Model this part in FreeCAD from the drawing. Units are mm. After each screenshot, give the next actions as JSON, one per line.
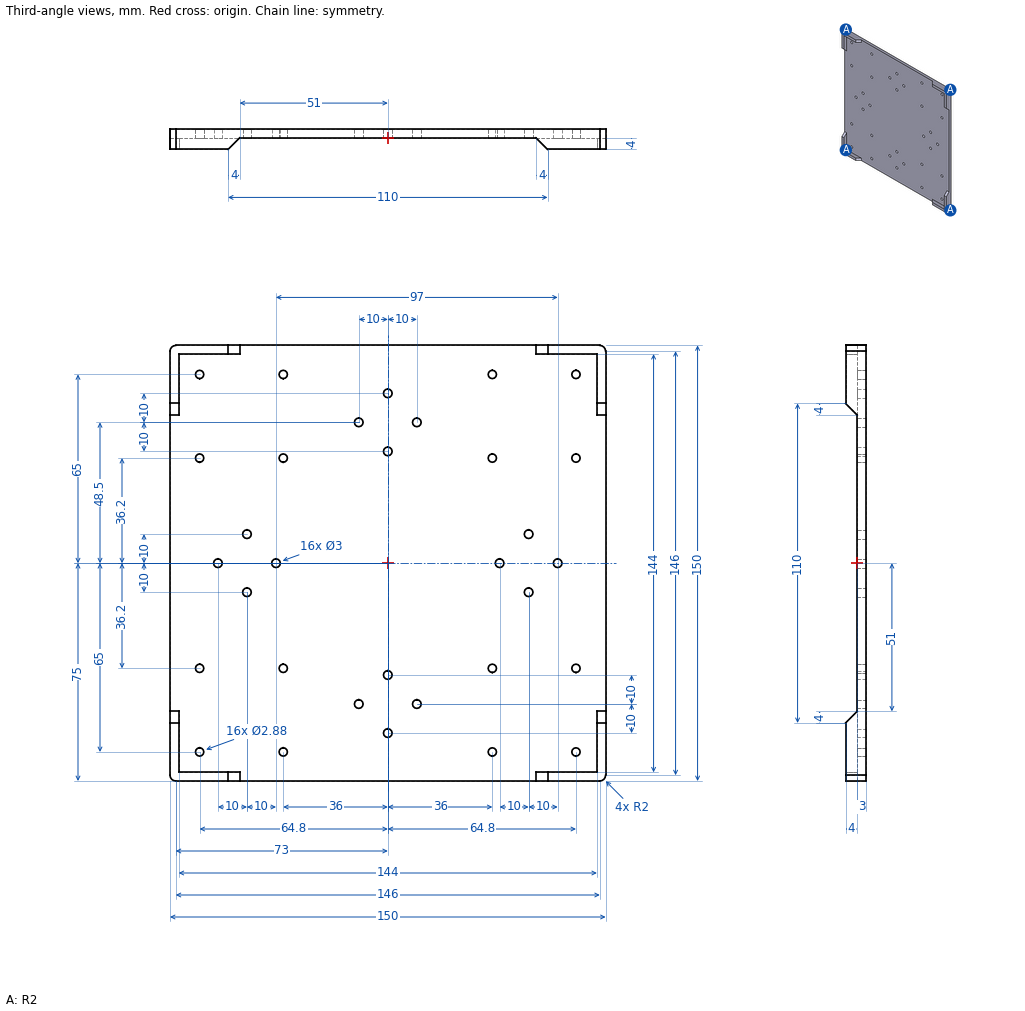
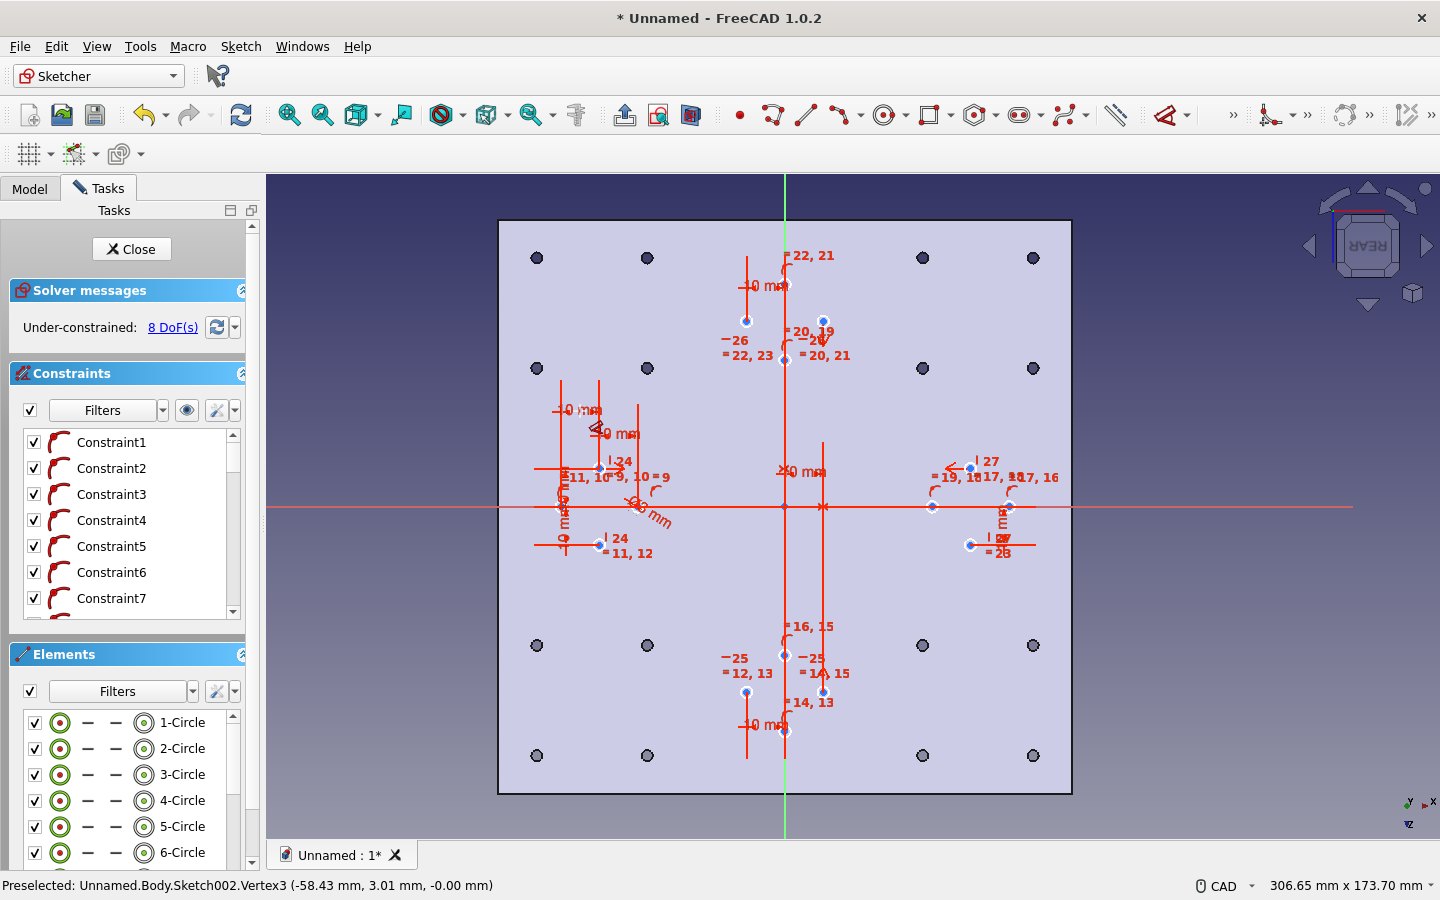
{"action": "left_click", "coordinate": [747, 692]}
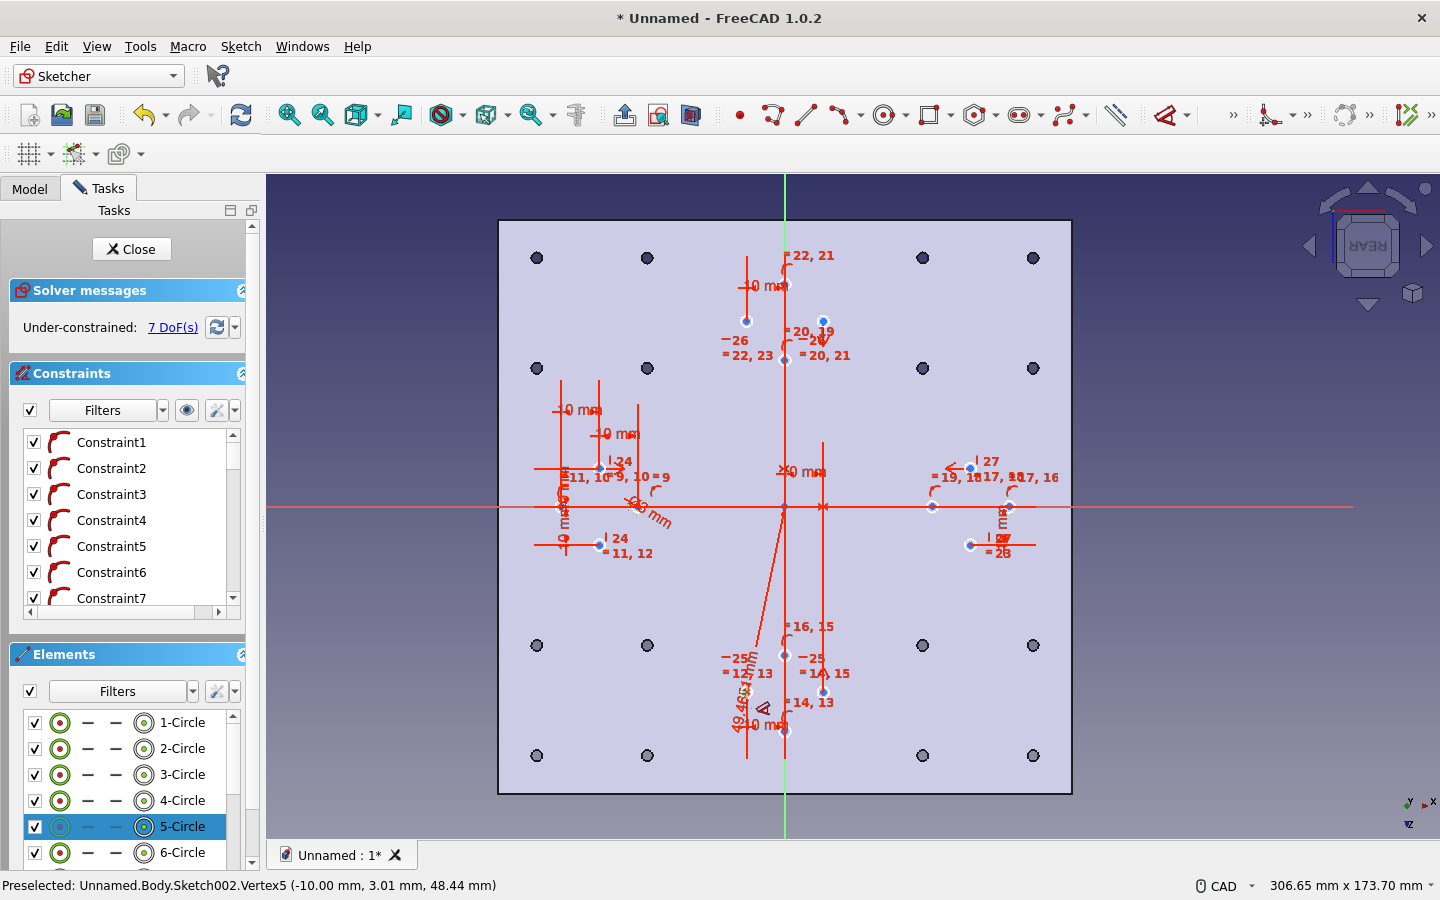
{"action": "left_click", "coordinate": [785, 732]}
{"action": "left_click", "coordinate": [713, 703]}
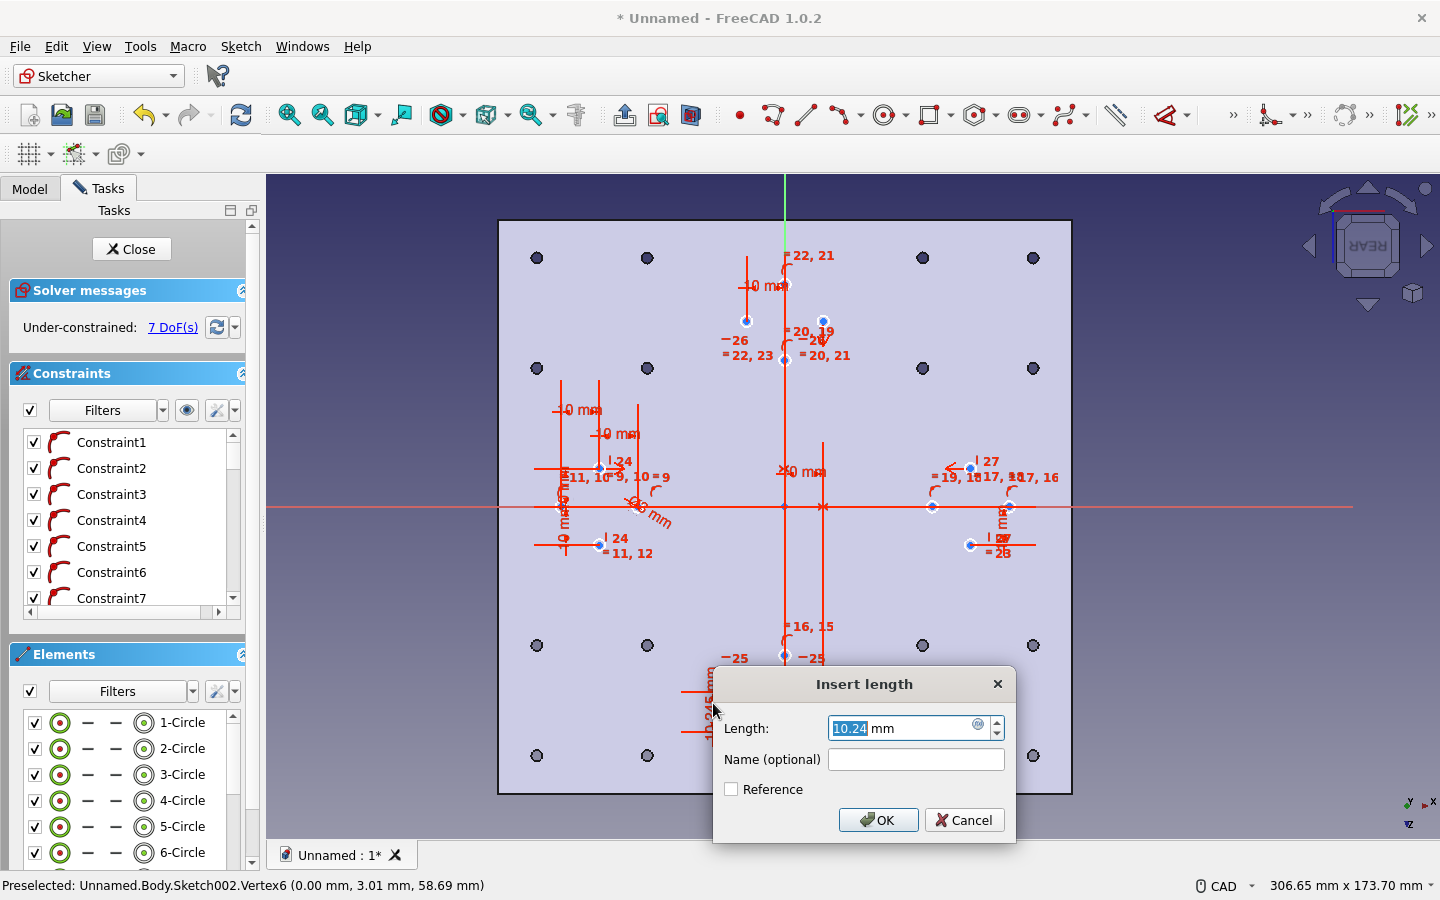
{"action": "type", "text": "10"}
{"action": "key", "text": "Return"}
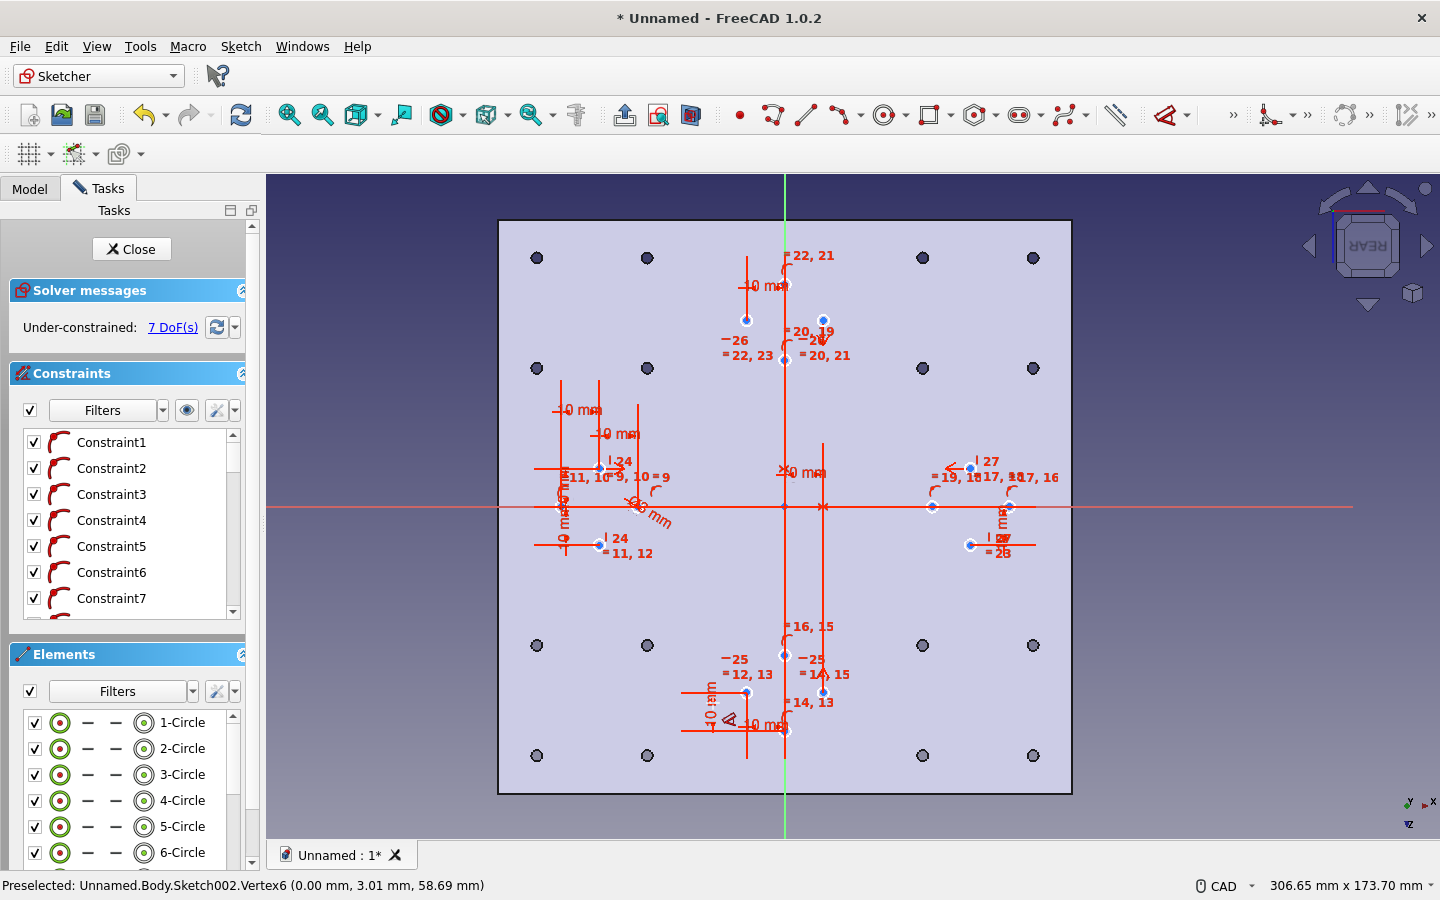
{"action": "left_click", "coordinate": [747, 693]}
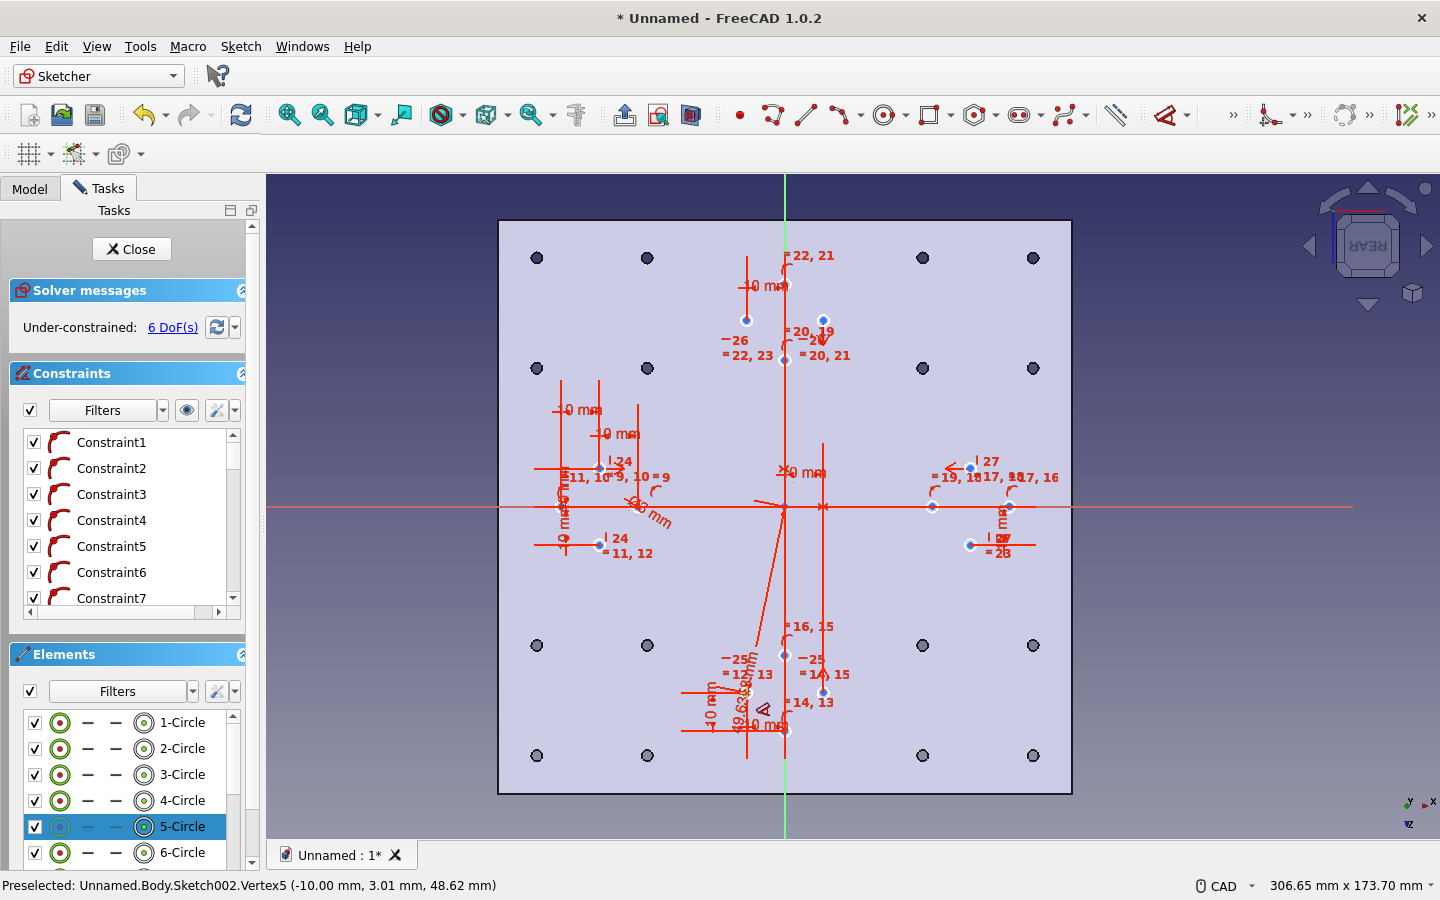
{"action": "left_click", "coordinate": [785, 656]}
{"action": "left_click", "coordinate": [713, 674]}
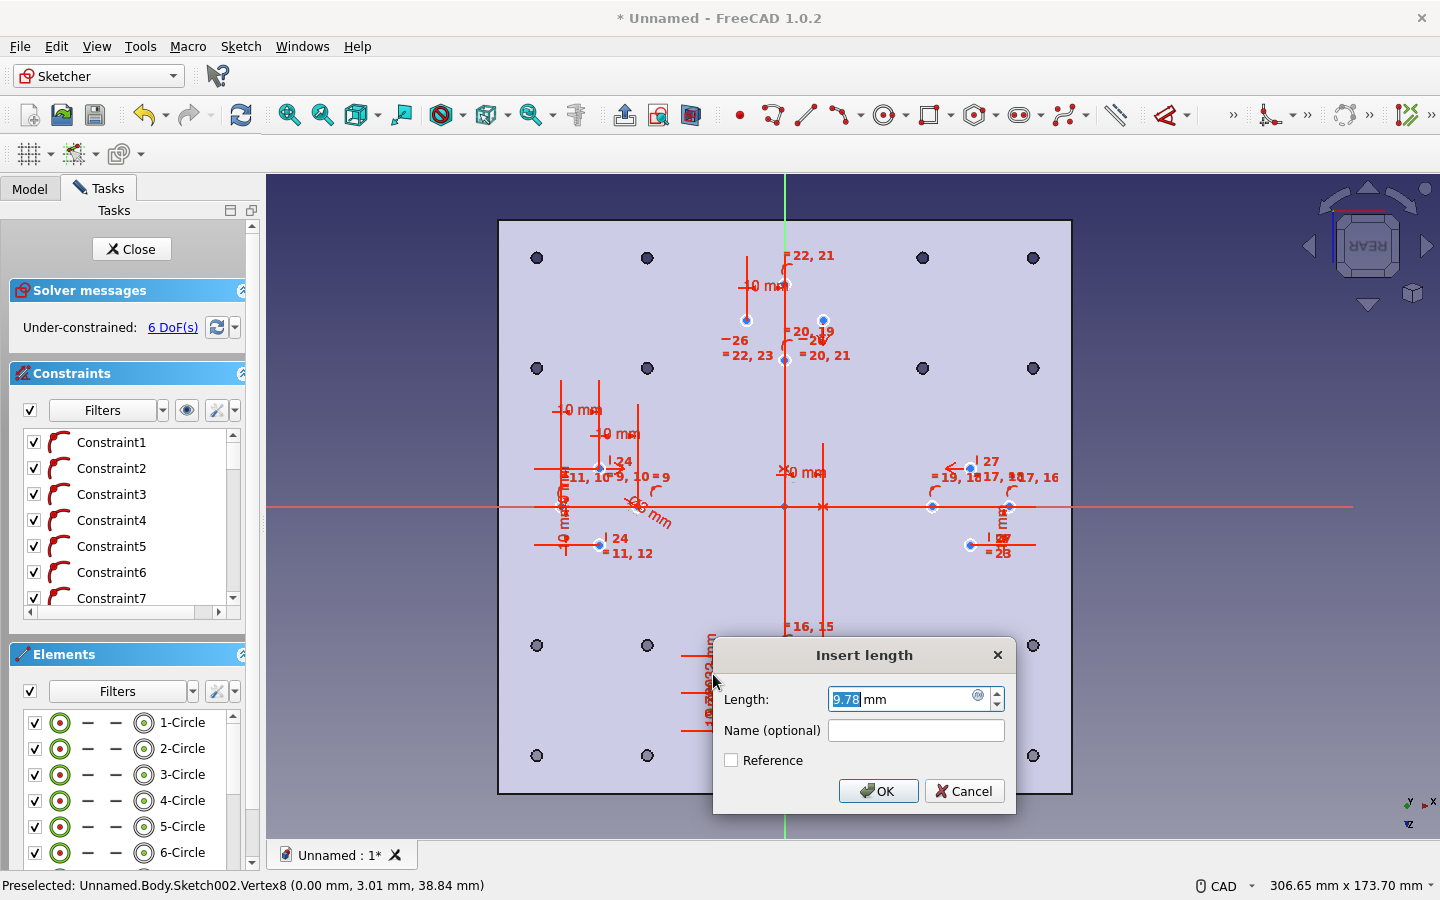
{"action": "type", "text": "10"}
{"action": "key", "text": "Return"}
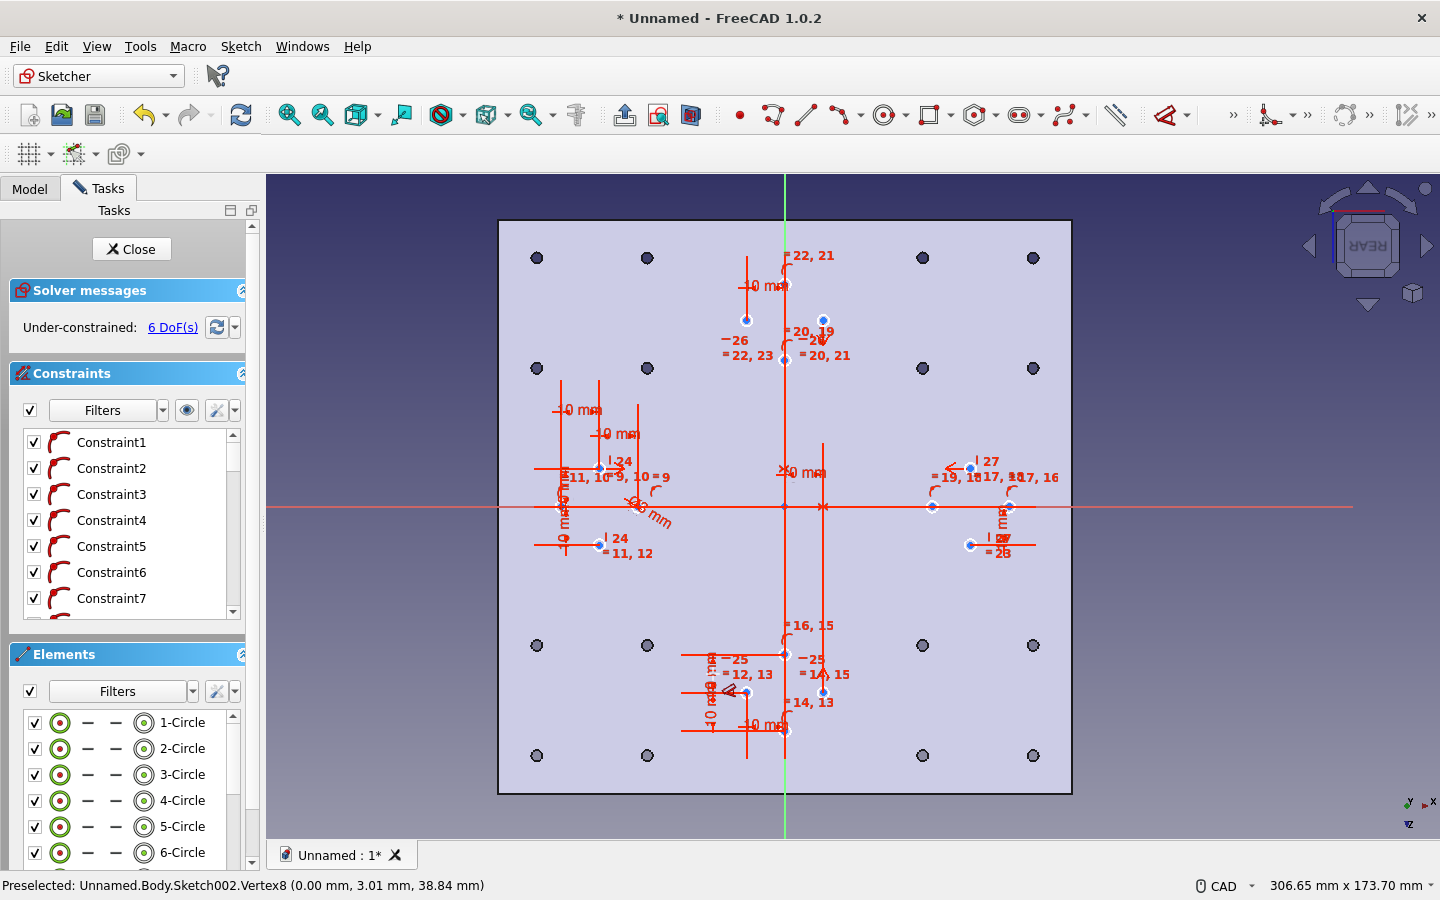
{"action": "left_click", "coordinate": [638, 507]}